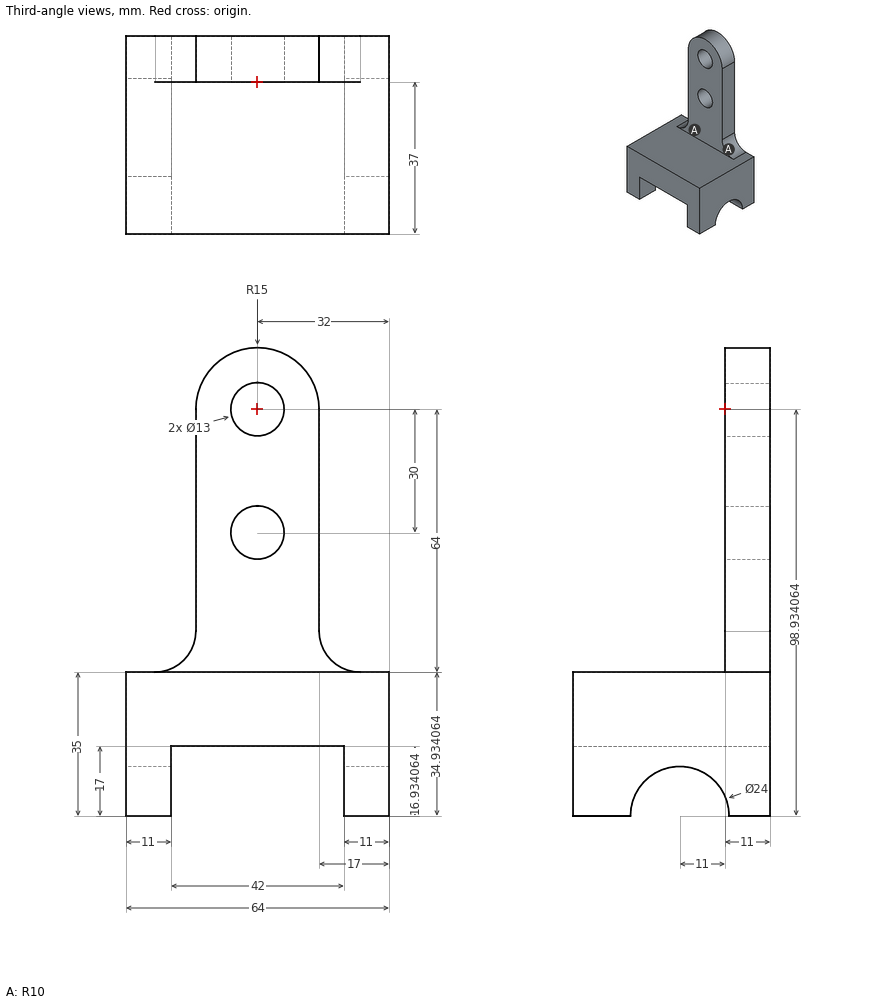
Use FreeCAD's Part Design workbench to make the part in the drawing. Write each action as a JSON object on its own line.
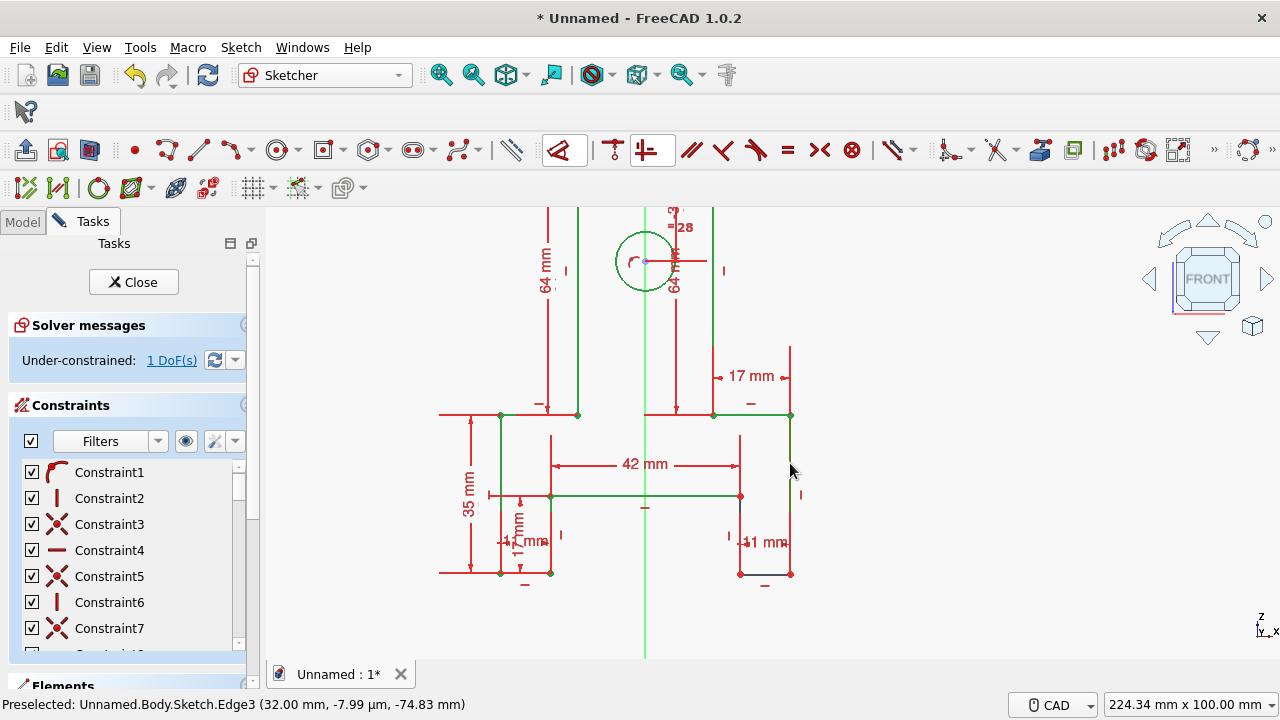
{"action": "key", "text": "i"}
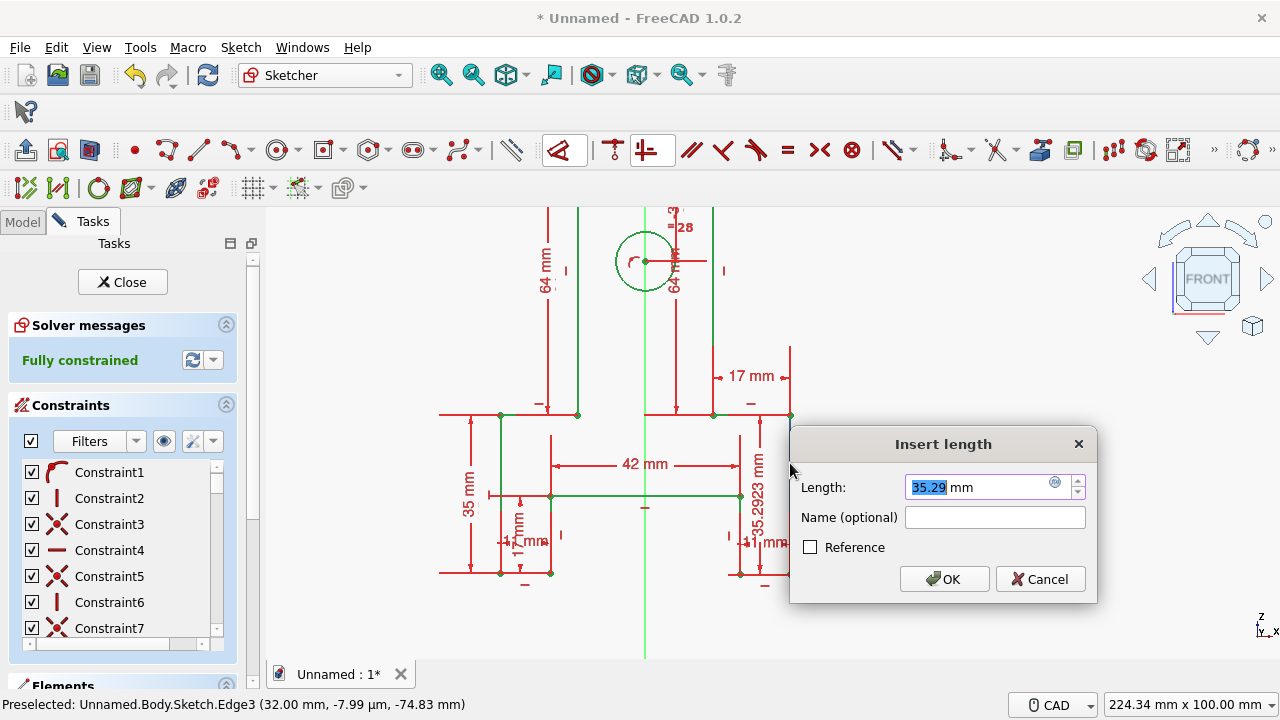
{"action": "type", "text": "34.934064"}
{"action": "key", "text": "Return"}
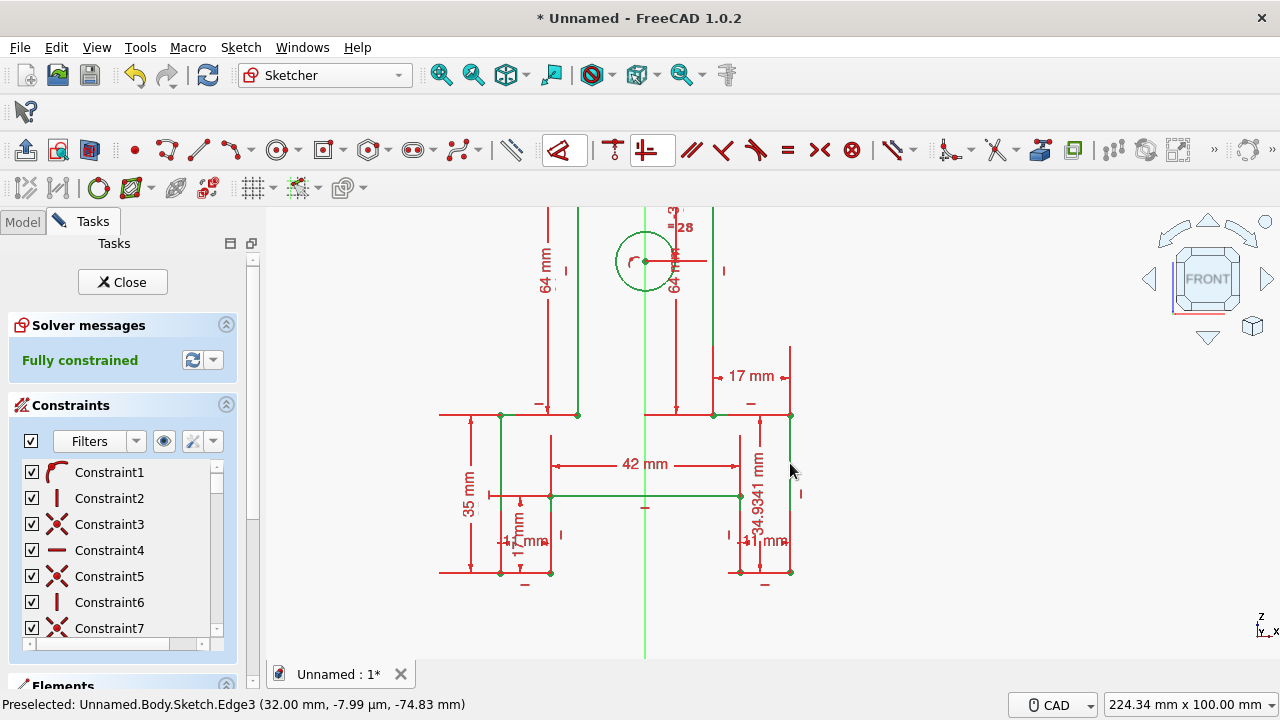
{"action": "left_click", "coordinate": [123, 282]}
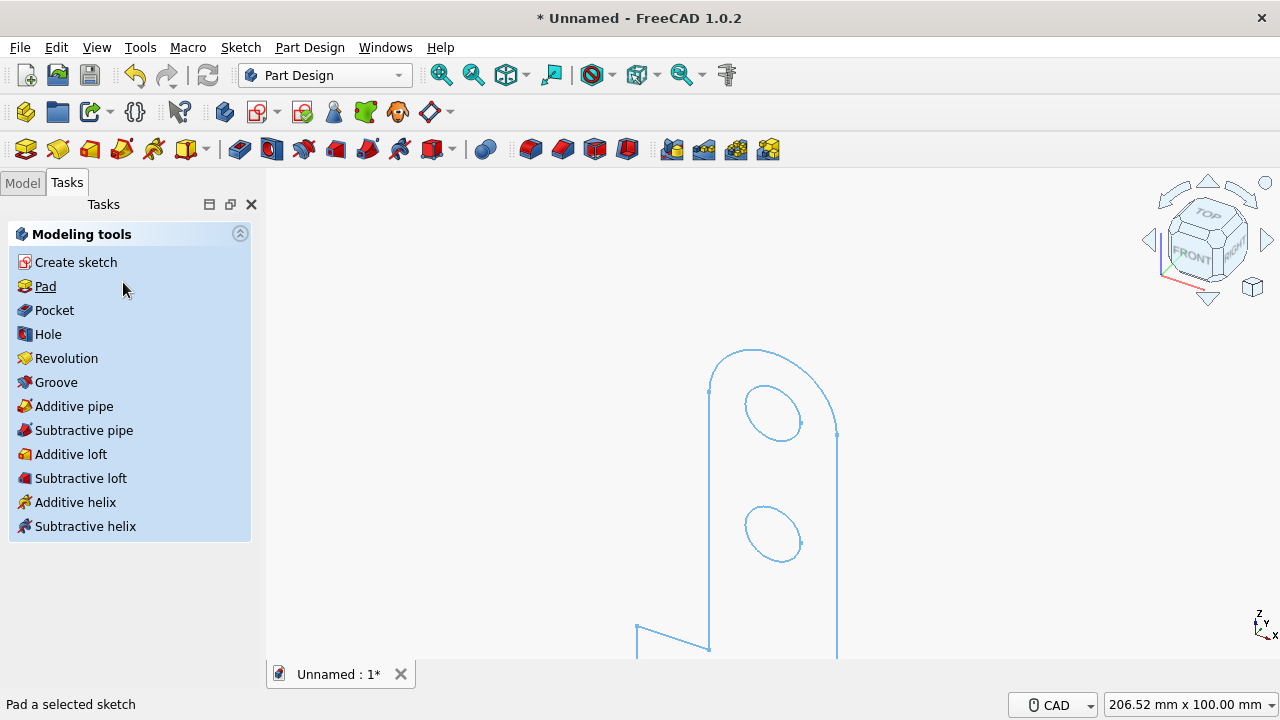
{"action": "left_click", "coordinate": [26, 150]}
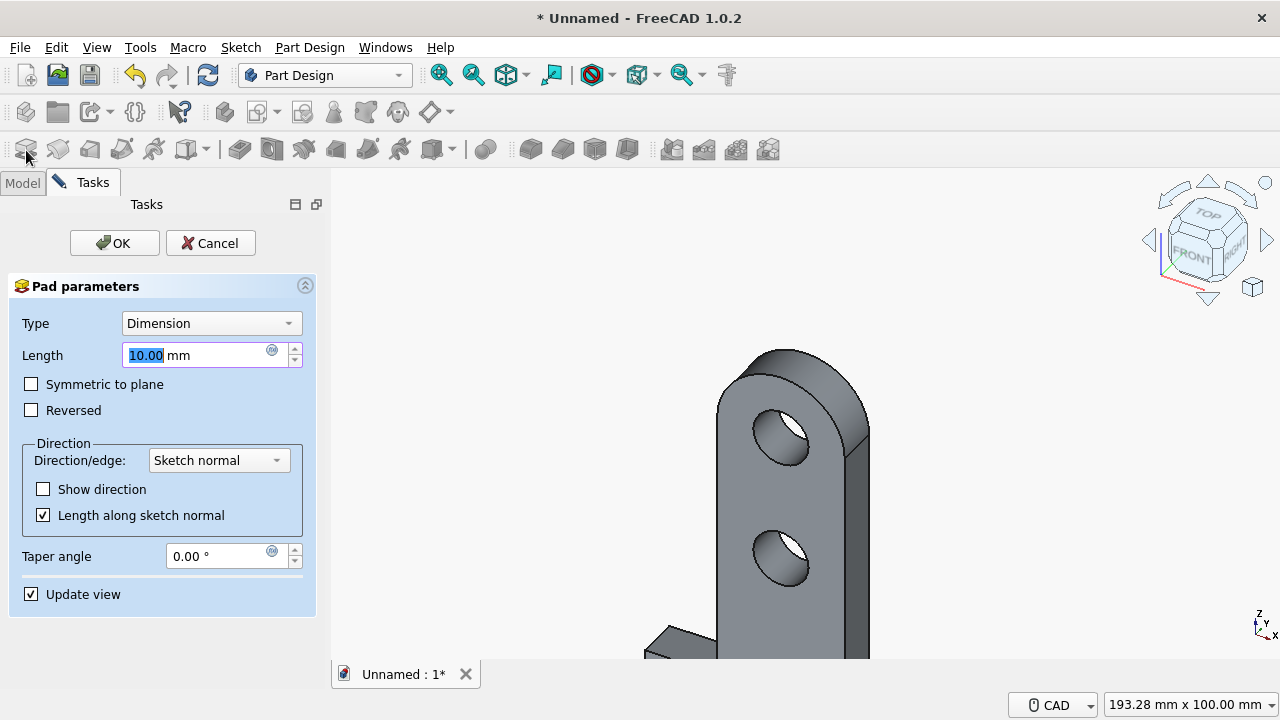
{"action": "type", "text": "11"}
{"action": "key", "text": "Tab"}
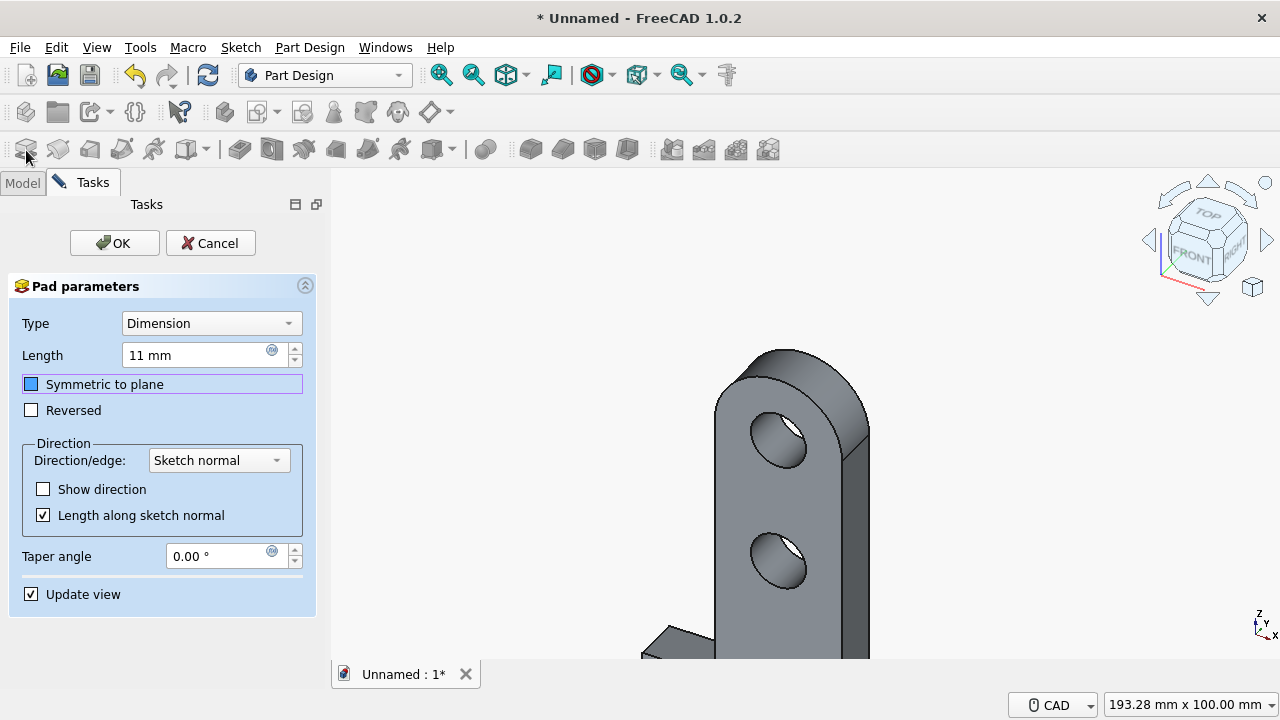
{"action": "left_click", "coordinate": [30, 410]}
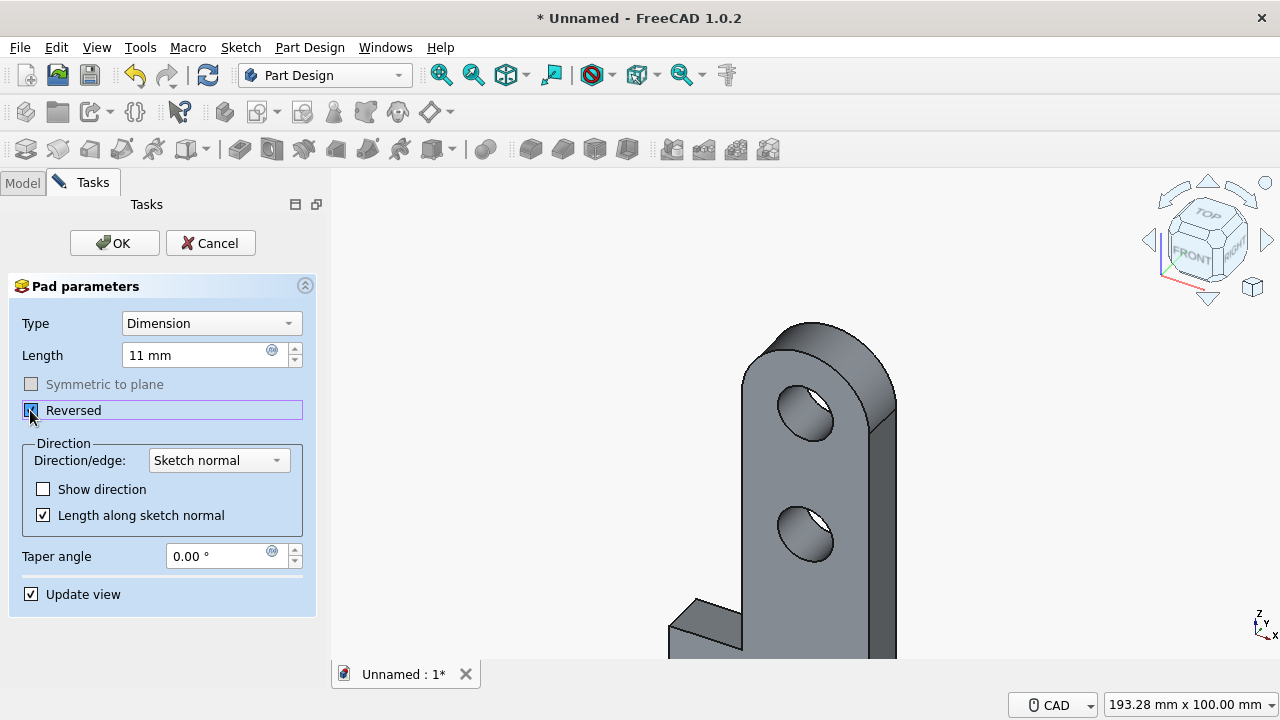
{"action": "left_click", "coordinate": [115, 243]}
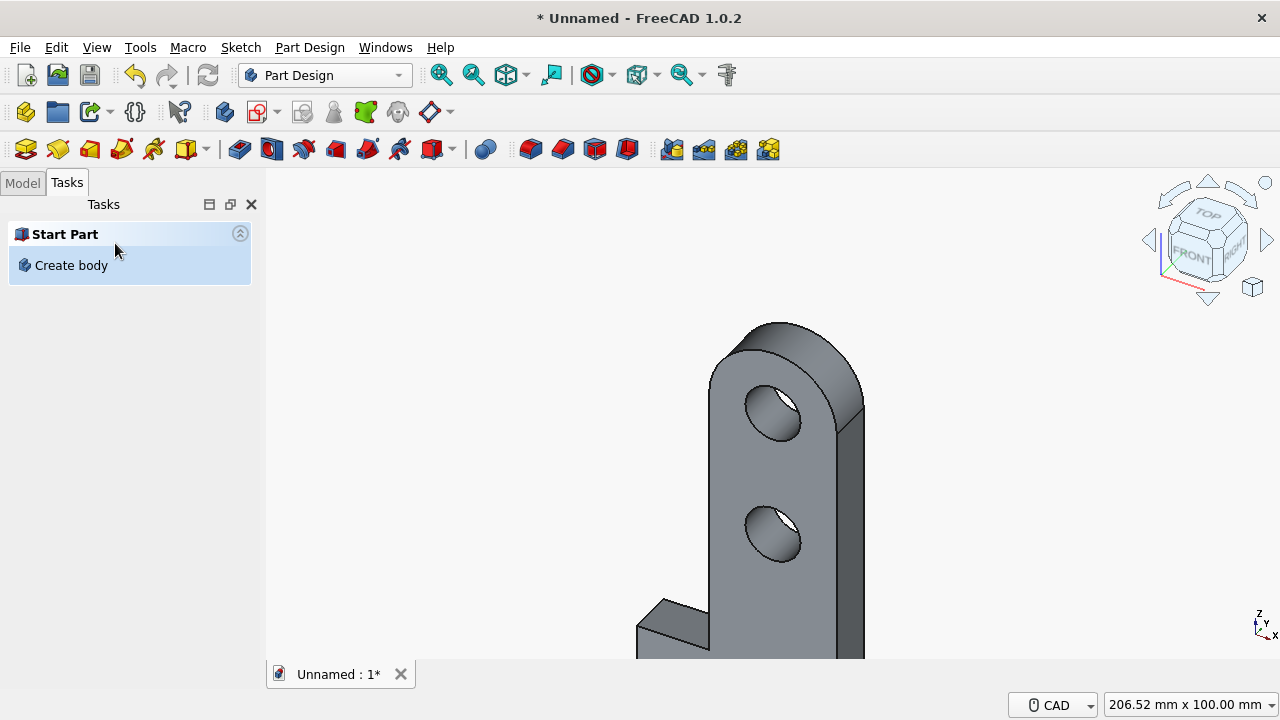
{"action": "left_click", "coordinate": [442, 76]}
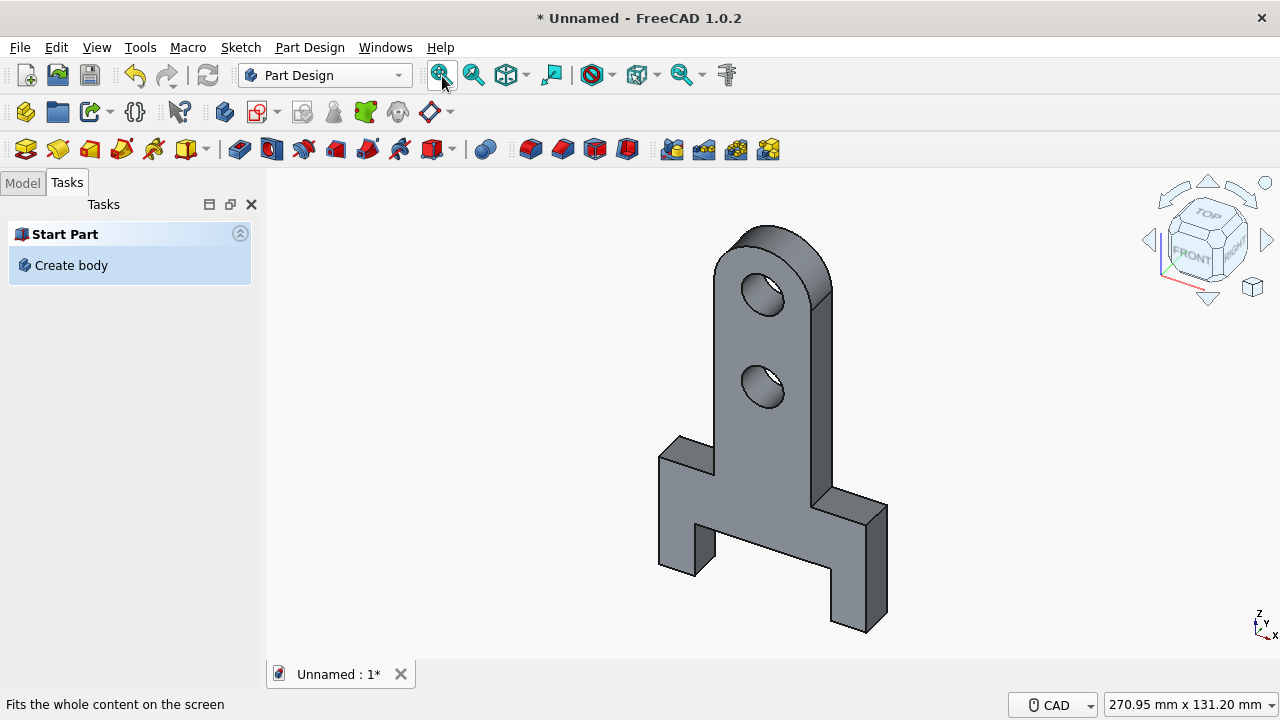
{"action": "left_click", "coordinate": [258, 112]}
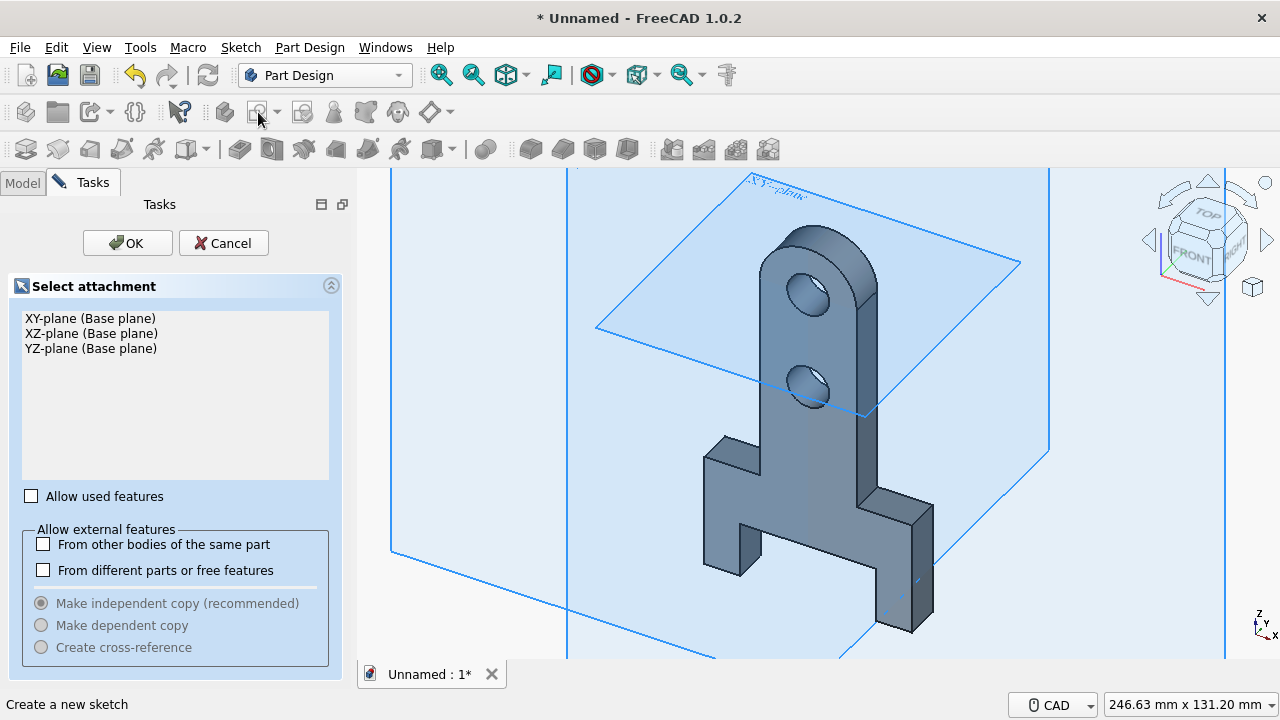
{"action": "left_click", "coordinate": [82, 334]}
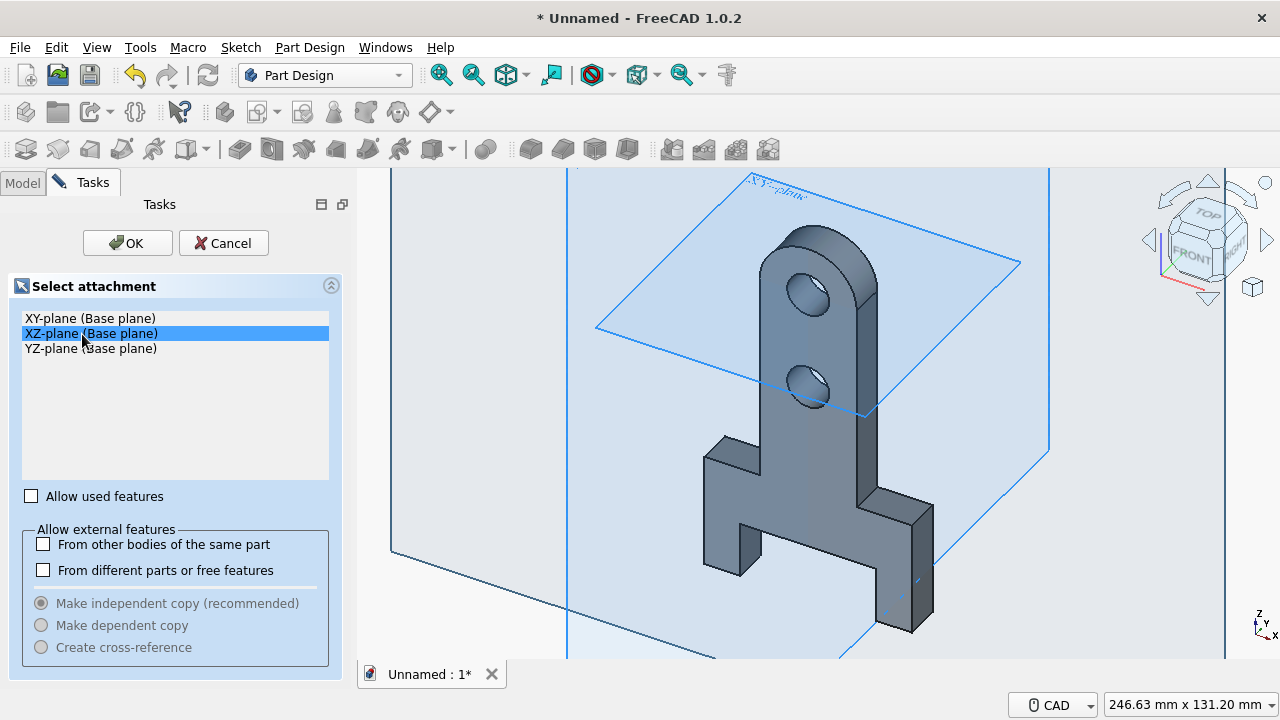
{"action": "left_click", "coordinate": [128, 243]}